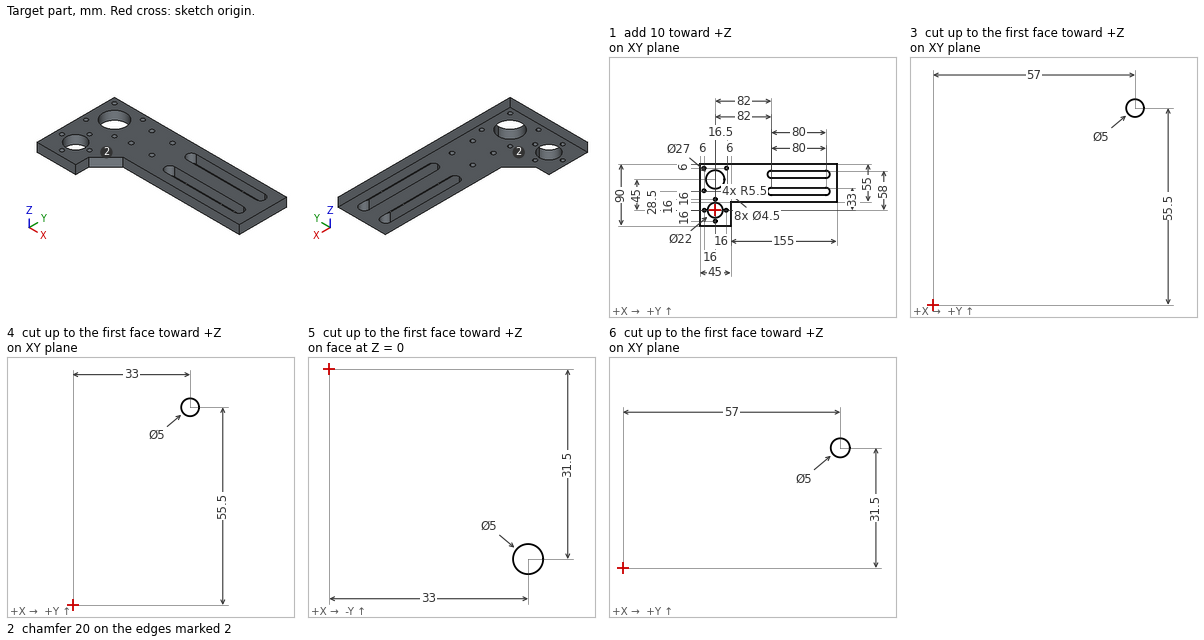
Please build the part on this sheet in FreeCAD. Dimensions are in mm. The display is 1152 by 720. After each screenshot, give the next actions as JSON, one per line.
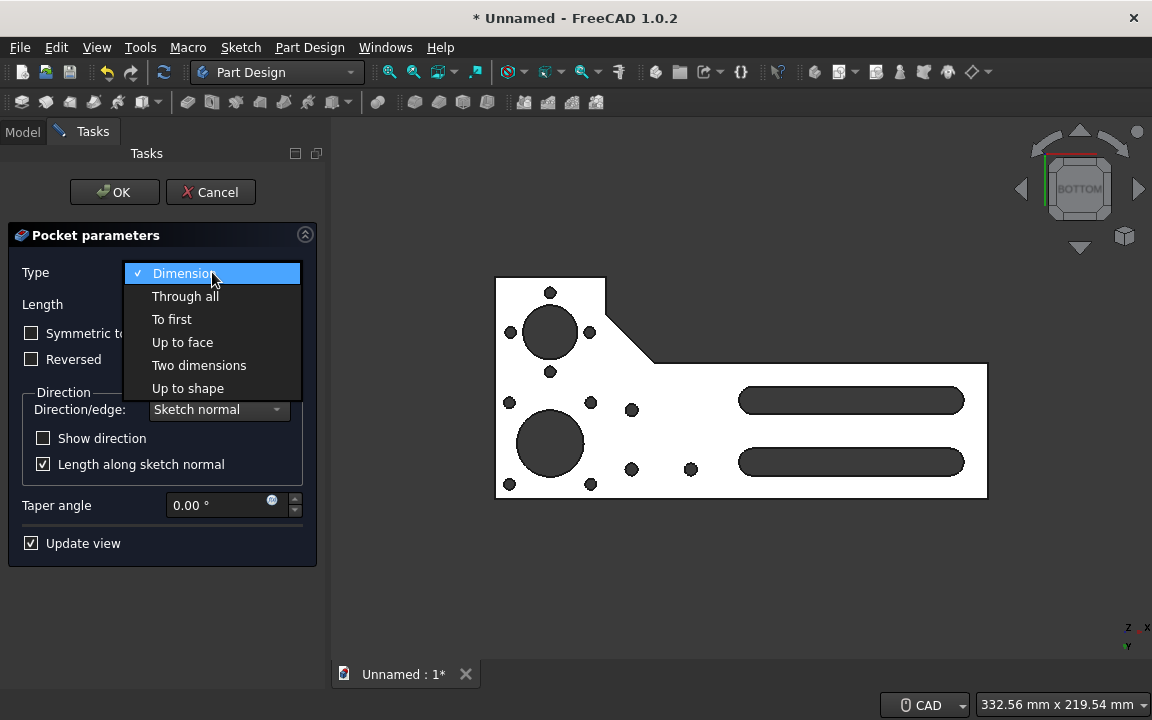
{"action": "left_click", "coordinate": [212, 320]}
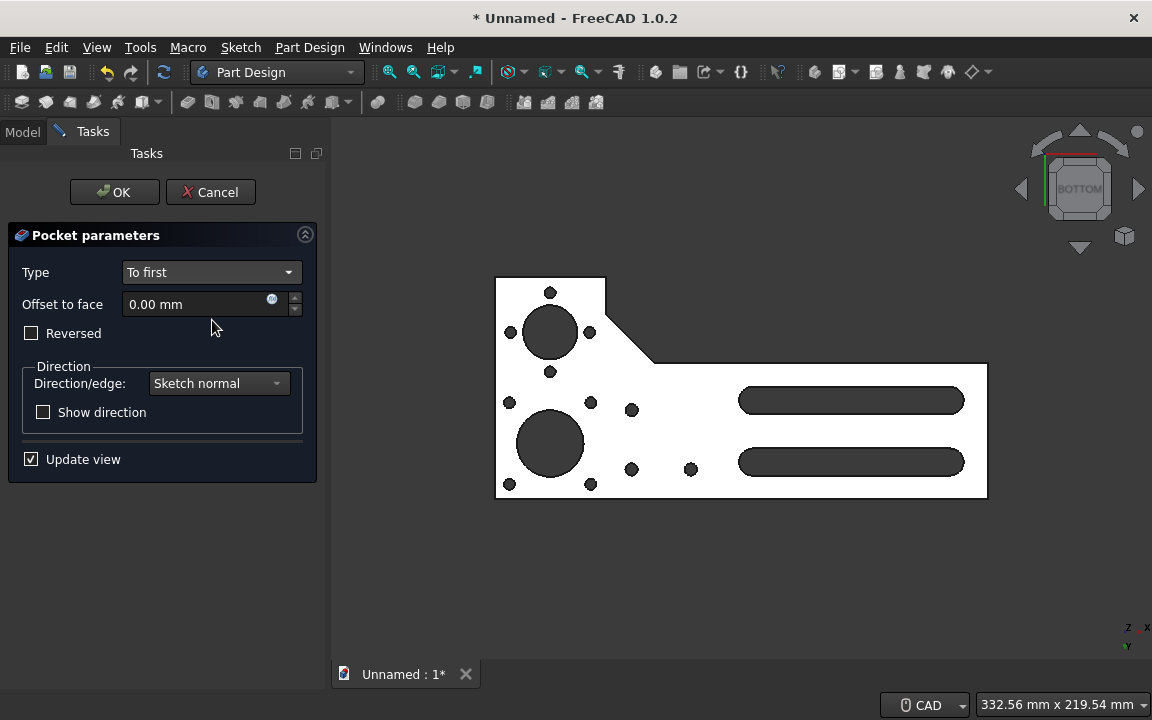
{"action": "left_click", "coordinate": [30, 333]}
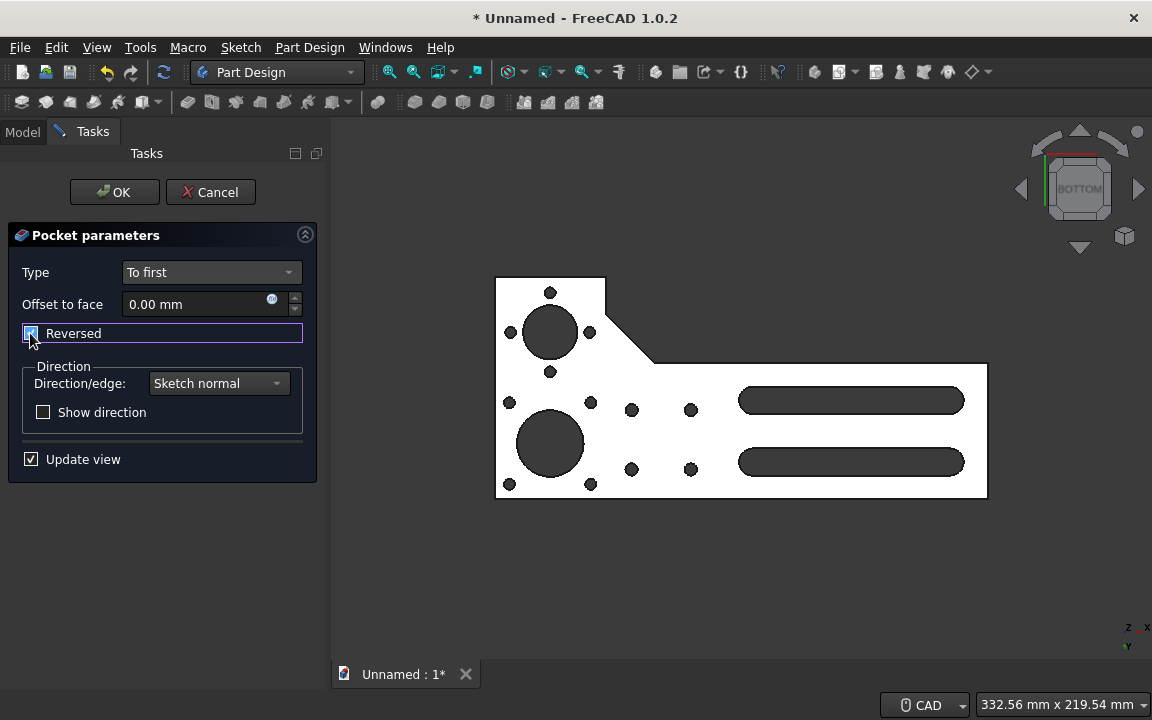
{"action": "left_click", "coordinate": [115, 192]}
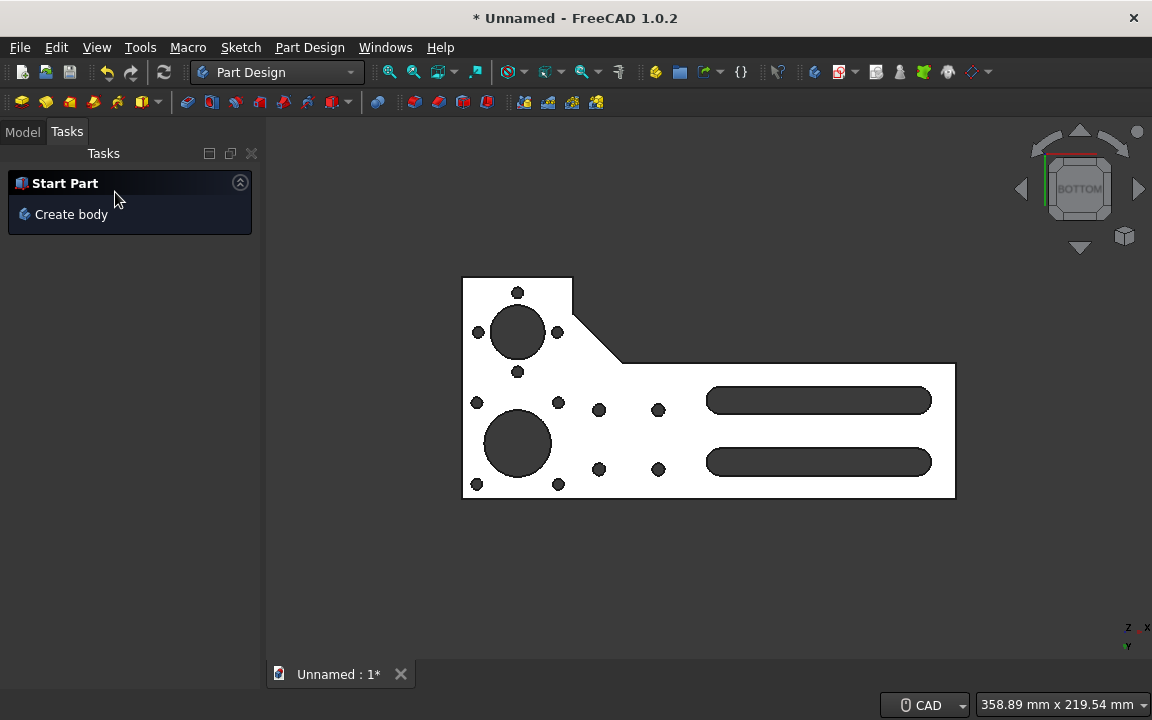
{"action": "key", "text": "0"}